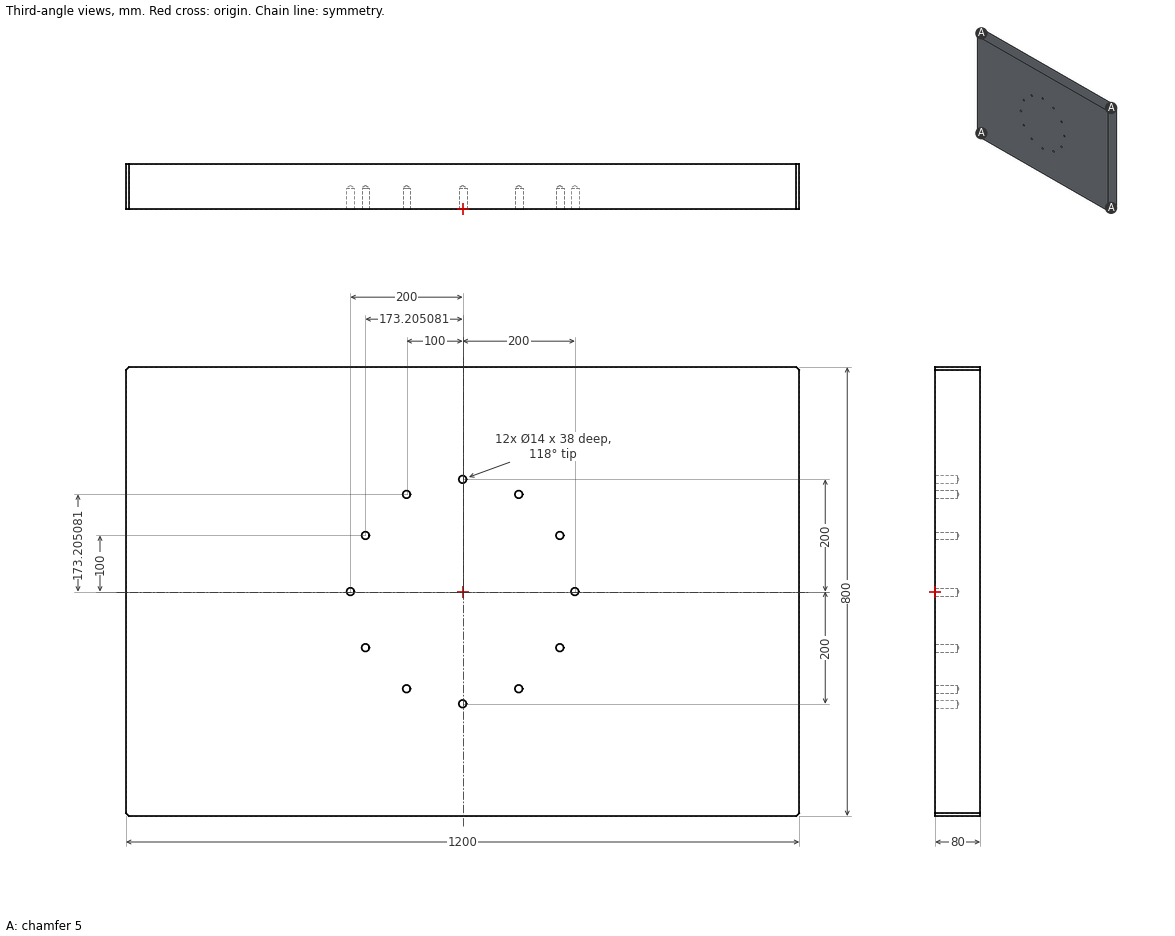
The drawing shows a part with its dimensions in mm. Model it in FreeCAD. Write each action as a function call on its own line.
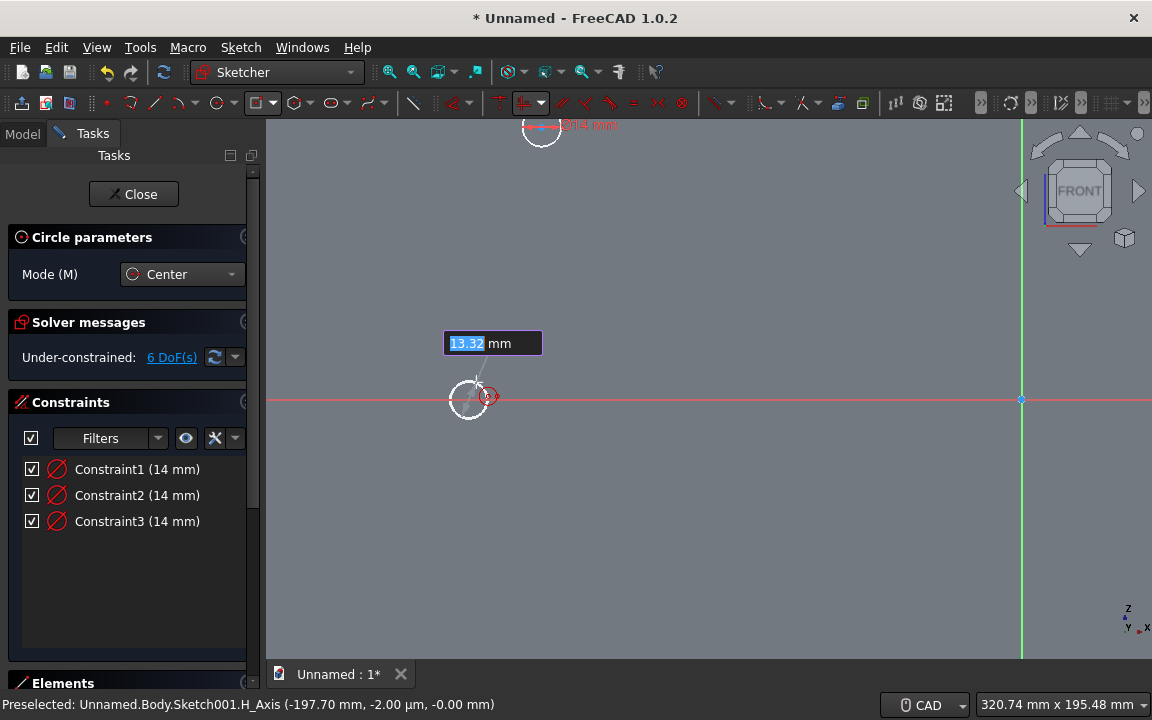
text(14)
key(Return)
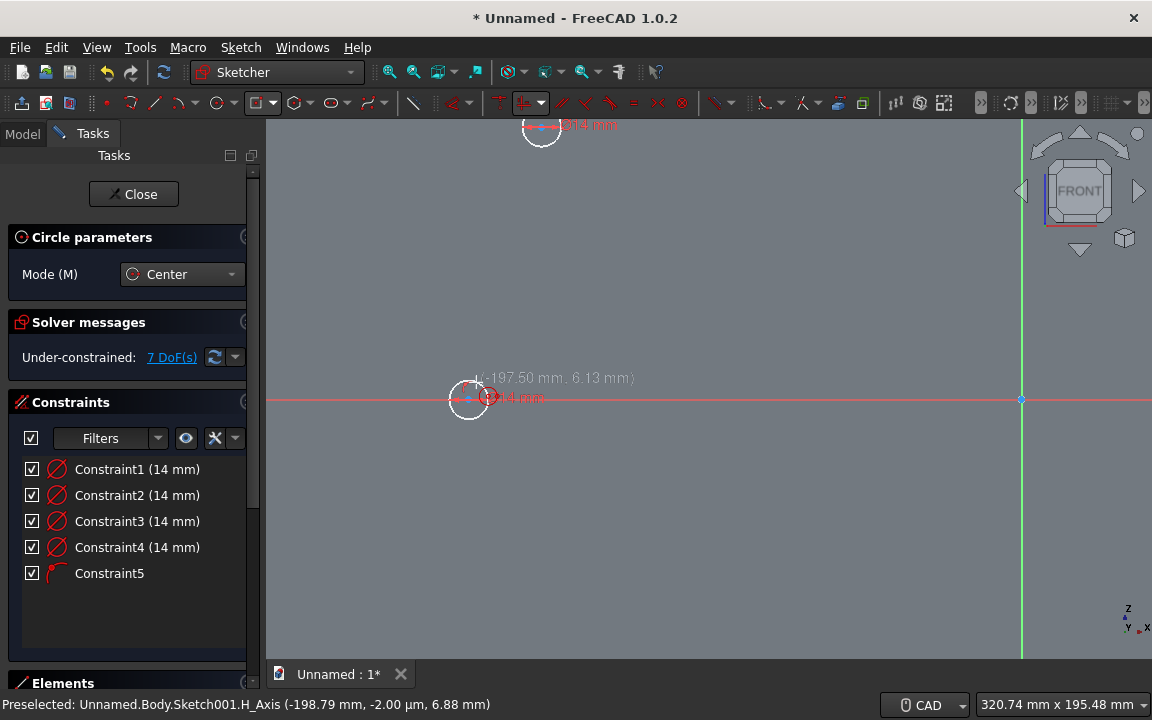
scroll(476, 384, down, 6)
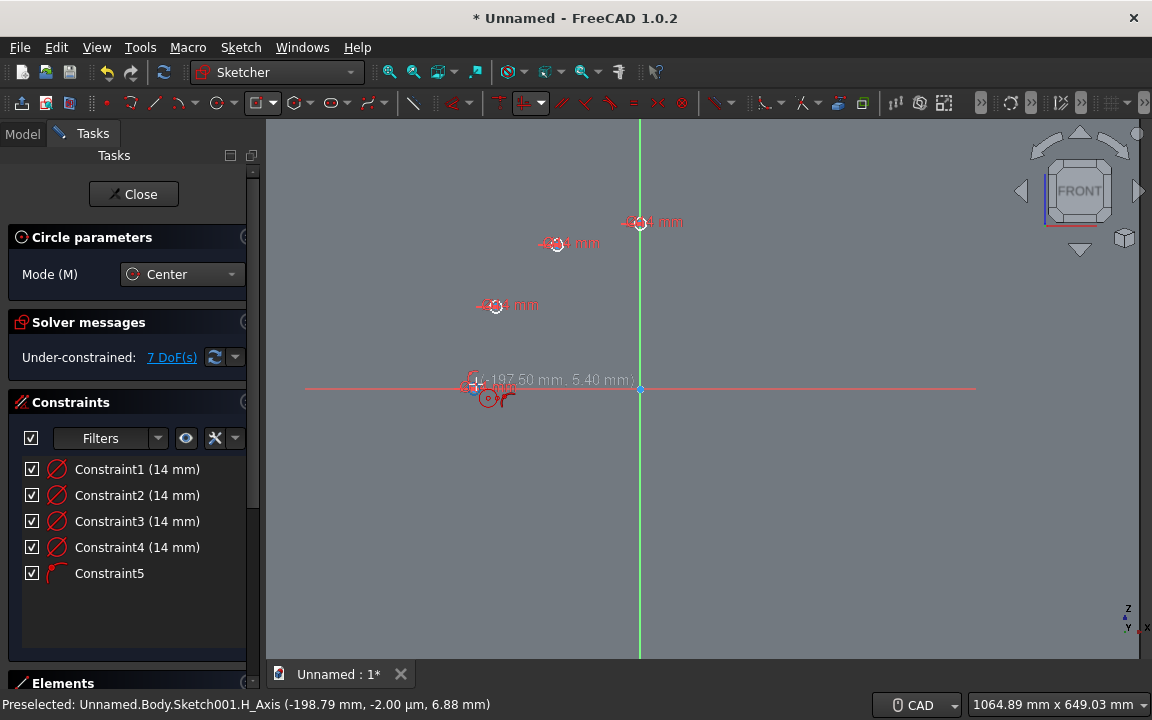
scroll(496, 472, up, 7)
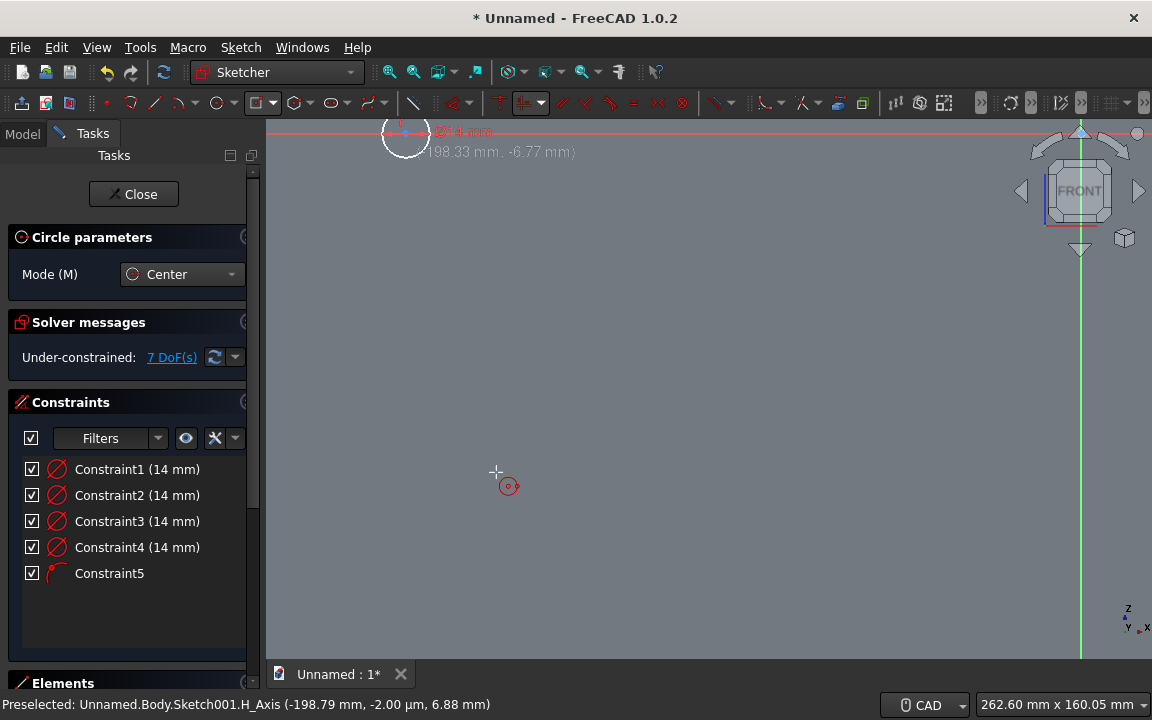
scroll(496, 472, down, 7)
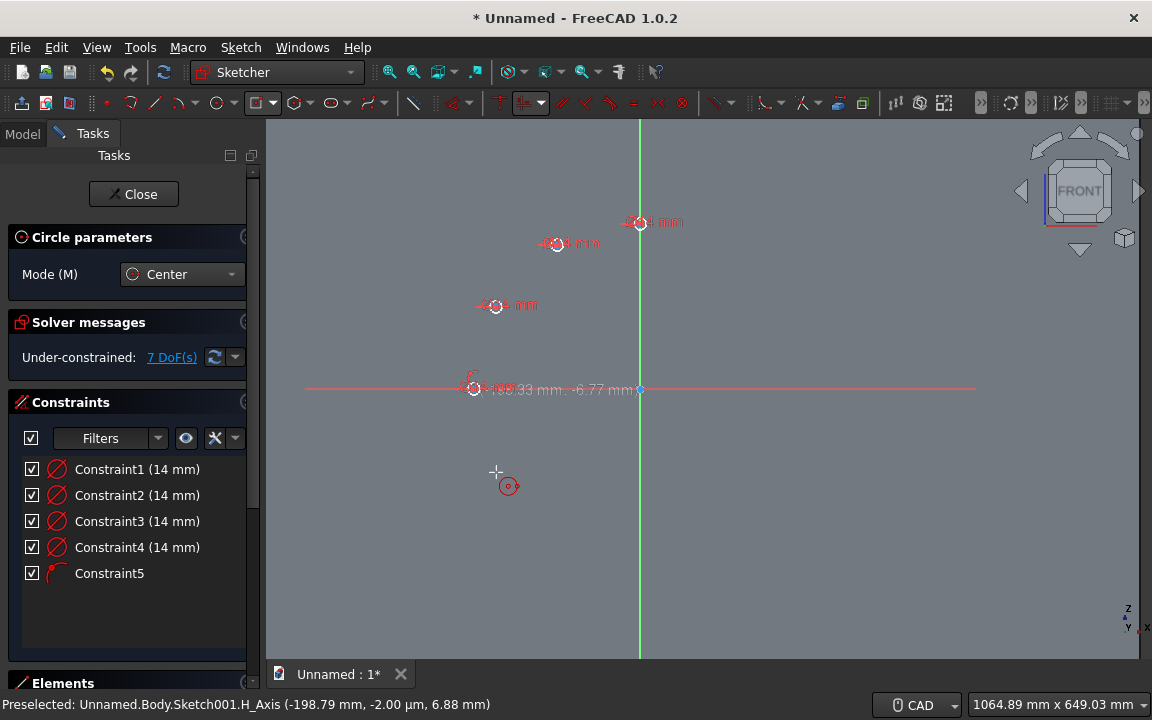
click(496, 472)
move(500, 468)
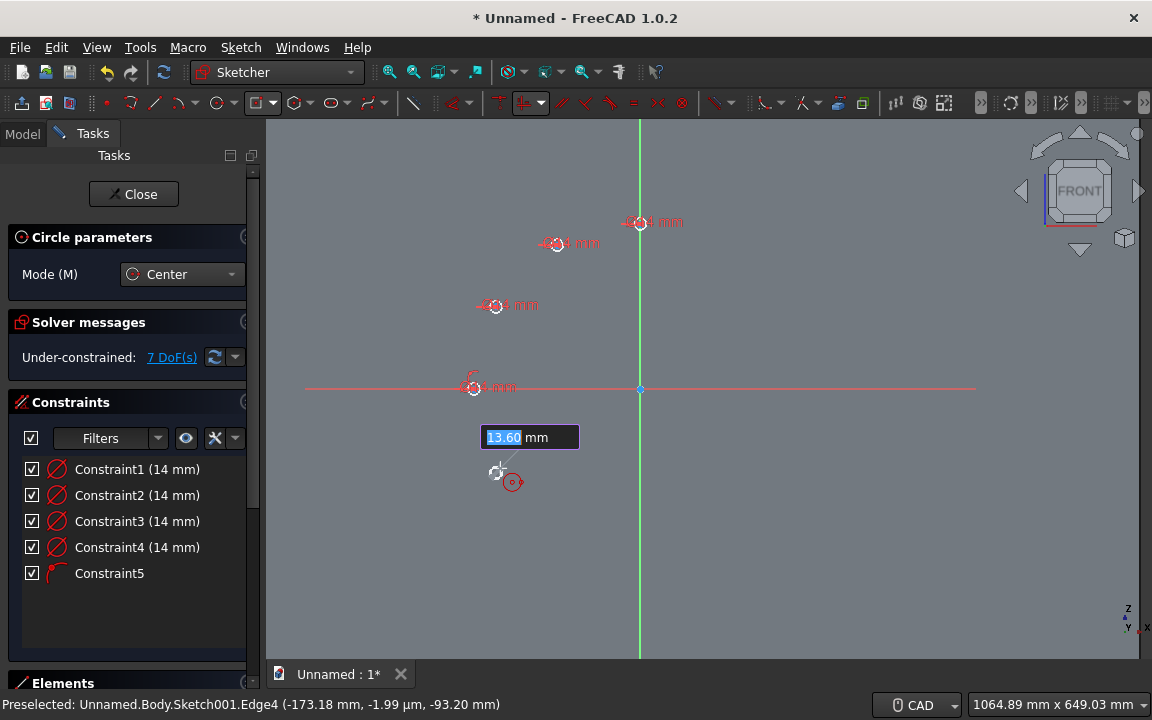
text(14)
key(Return)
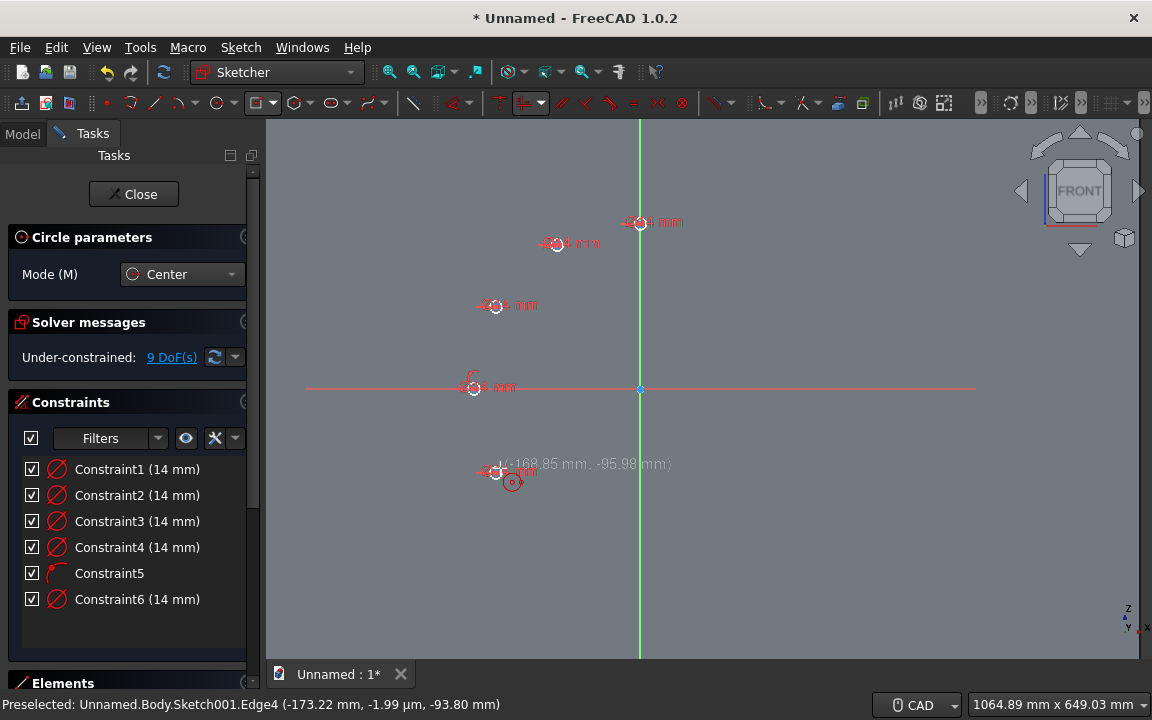
scroll(557, 533, up, 7)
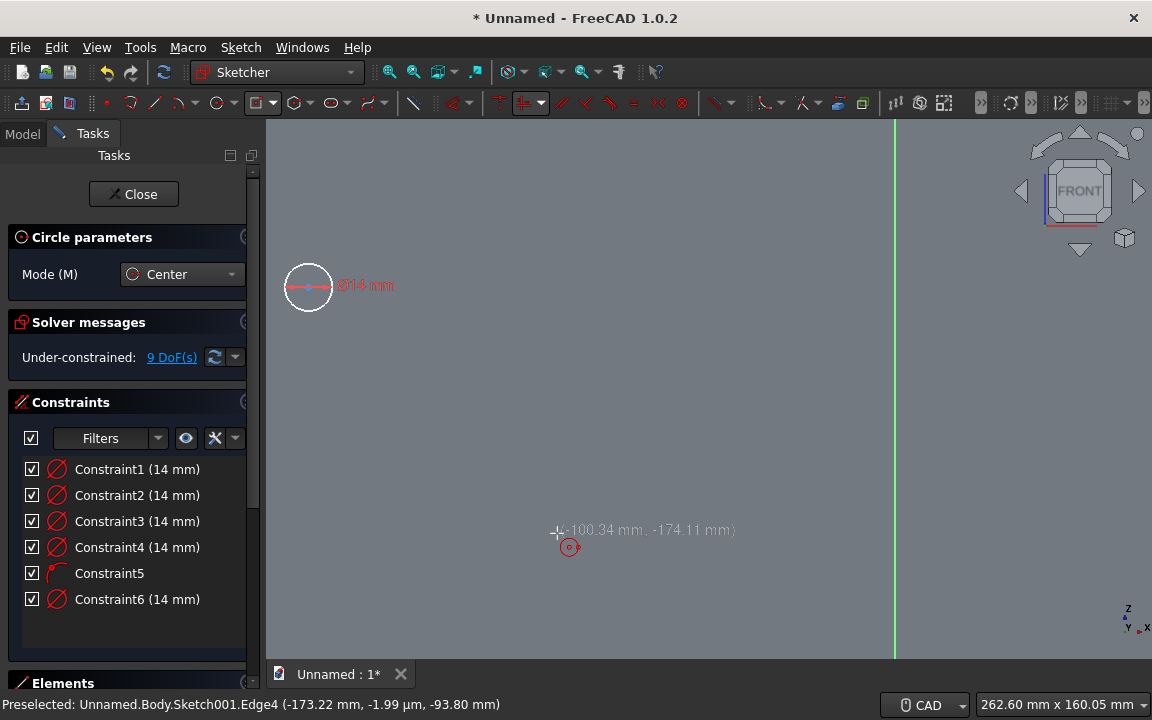
scroll(557, 534, down, 7)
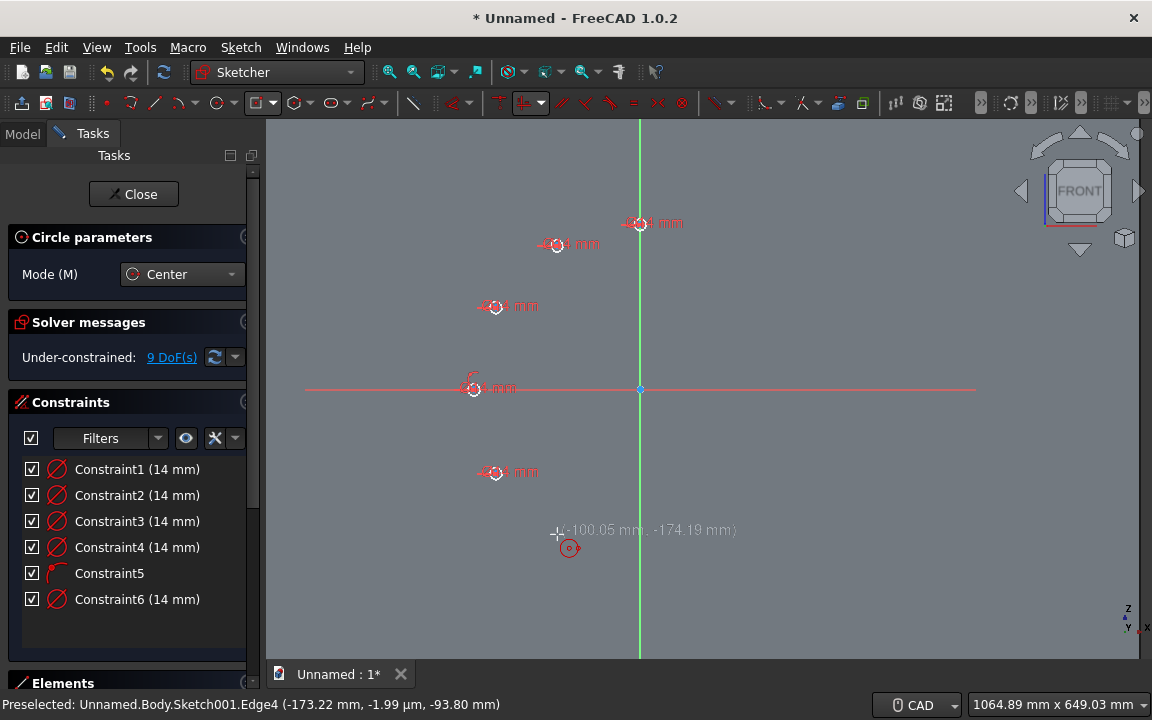
click(557, 534)
move(561, 530)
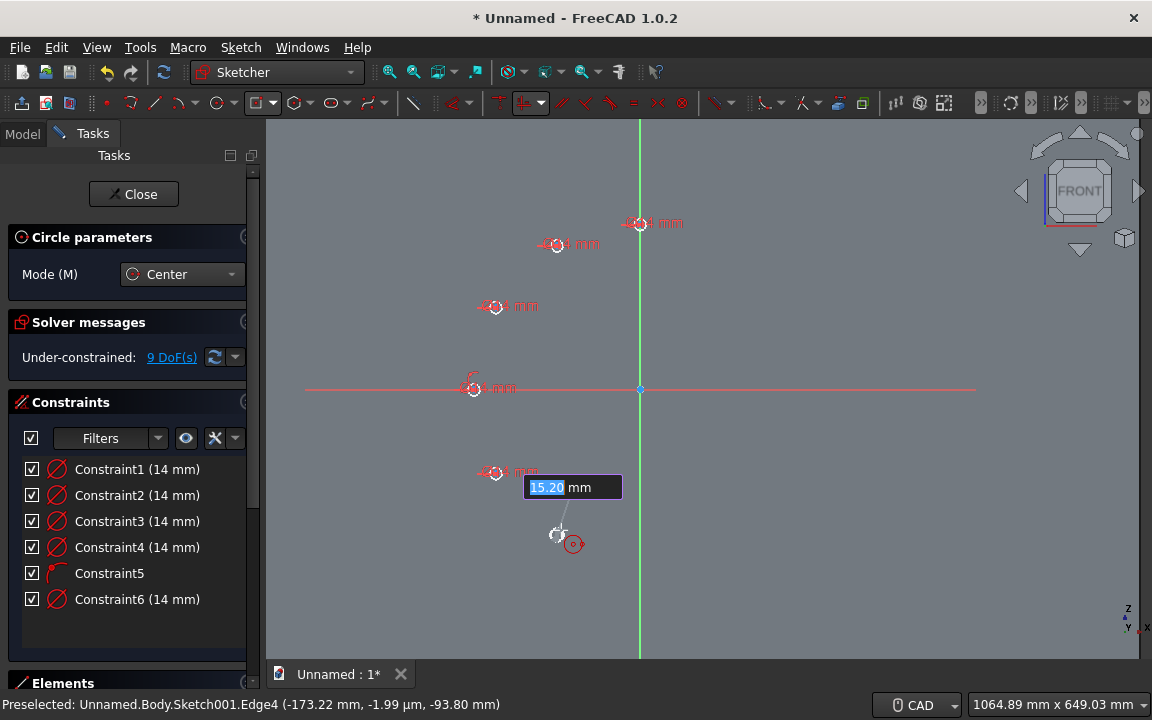
text(14)
key(Return)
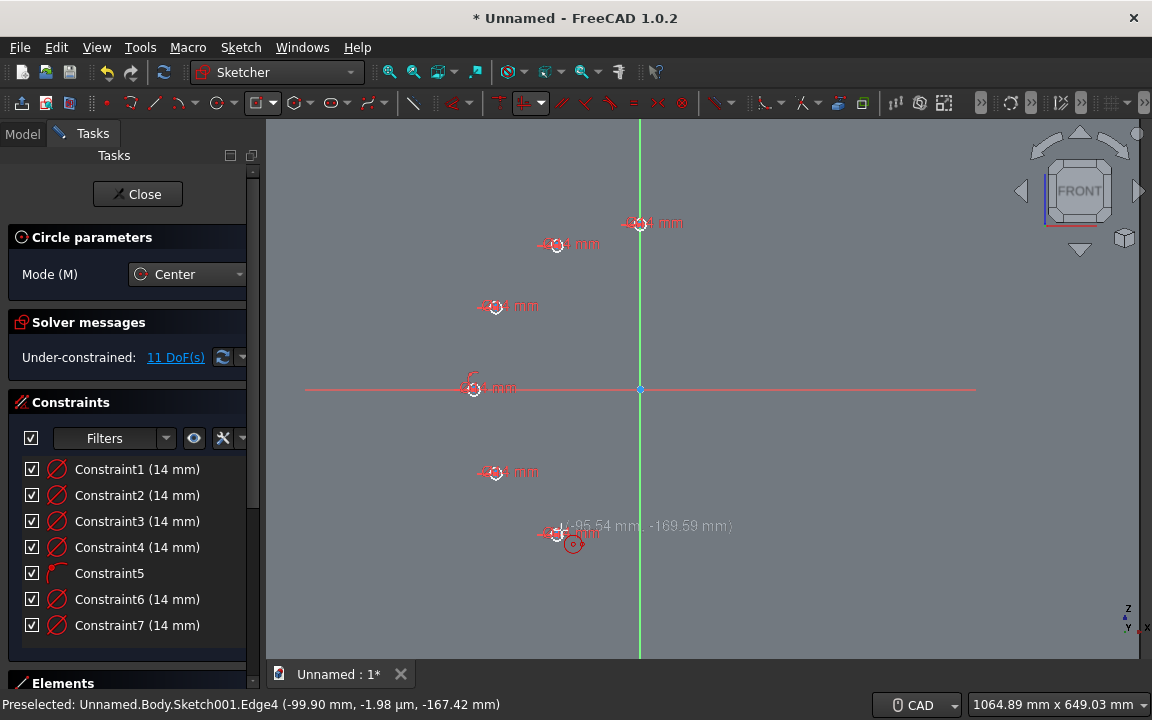
scroll(640, 556, up, 7)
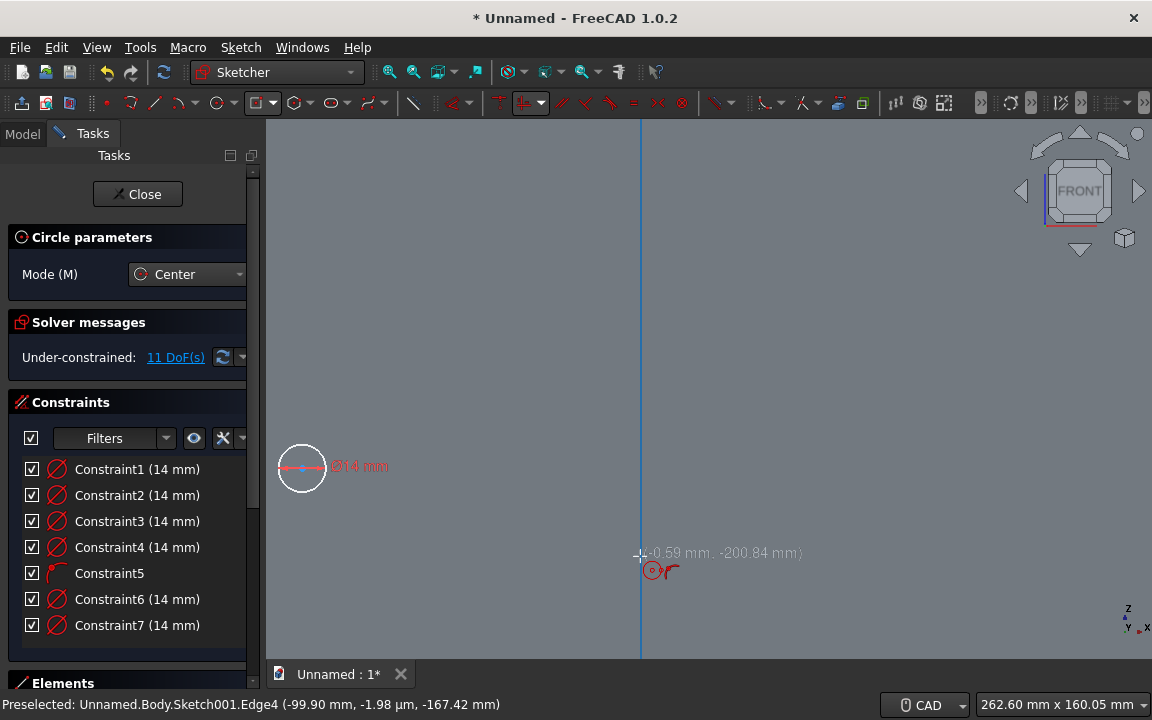
scroll(640, 556, down, 7)